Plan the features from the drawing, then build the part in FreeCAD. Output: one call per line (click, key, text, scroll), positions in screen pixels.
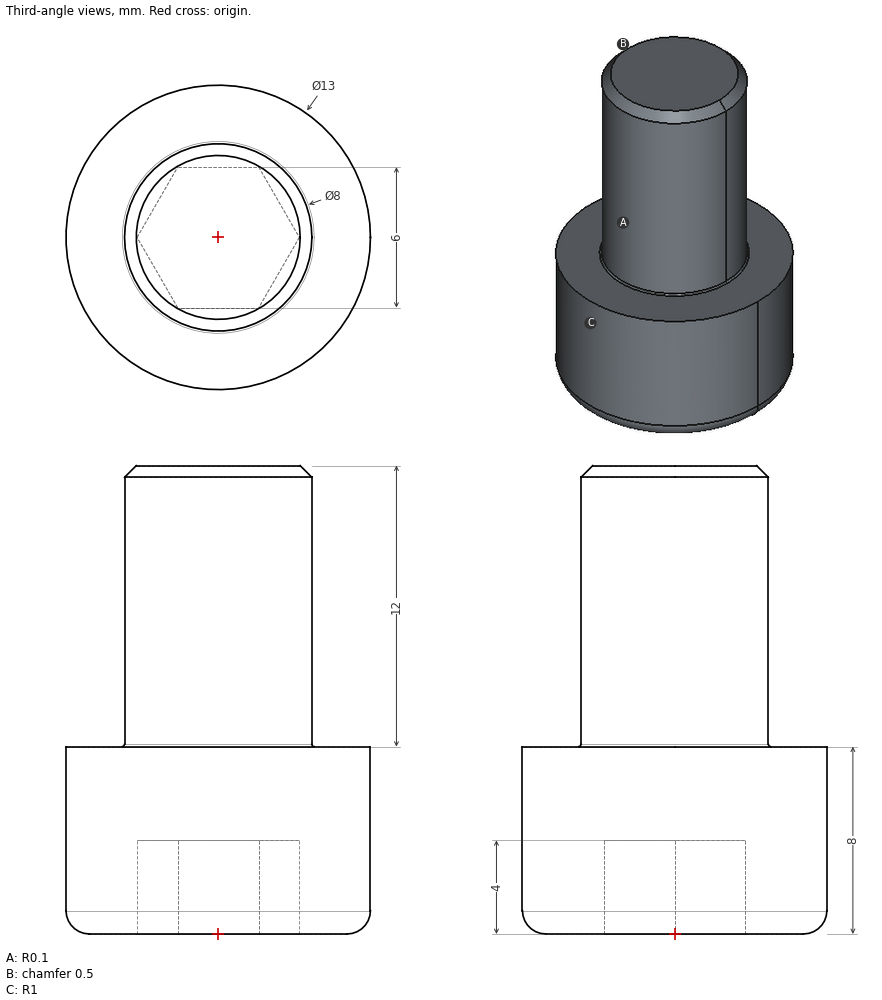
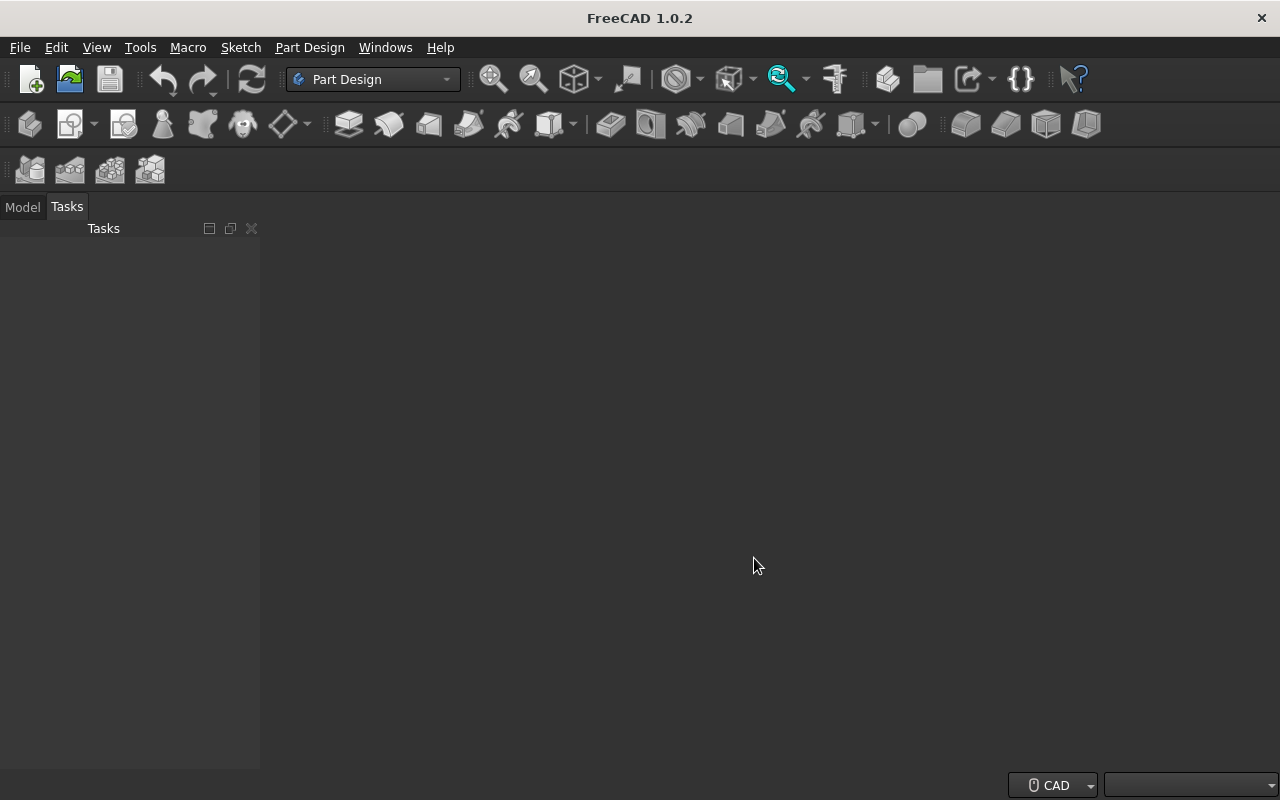
click(30, 80)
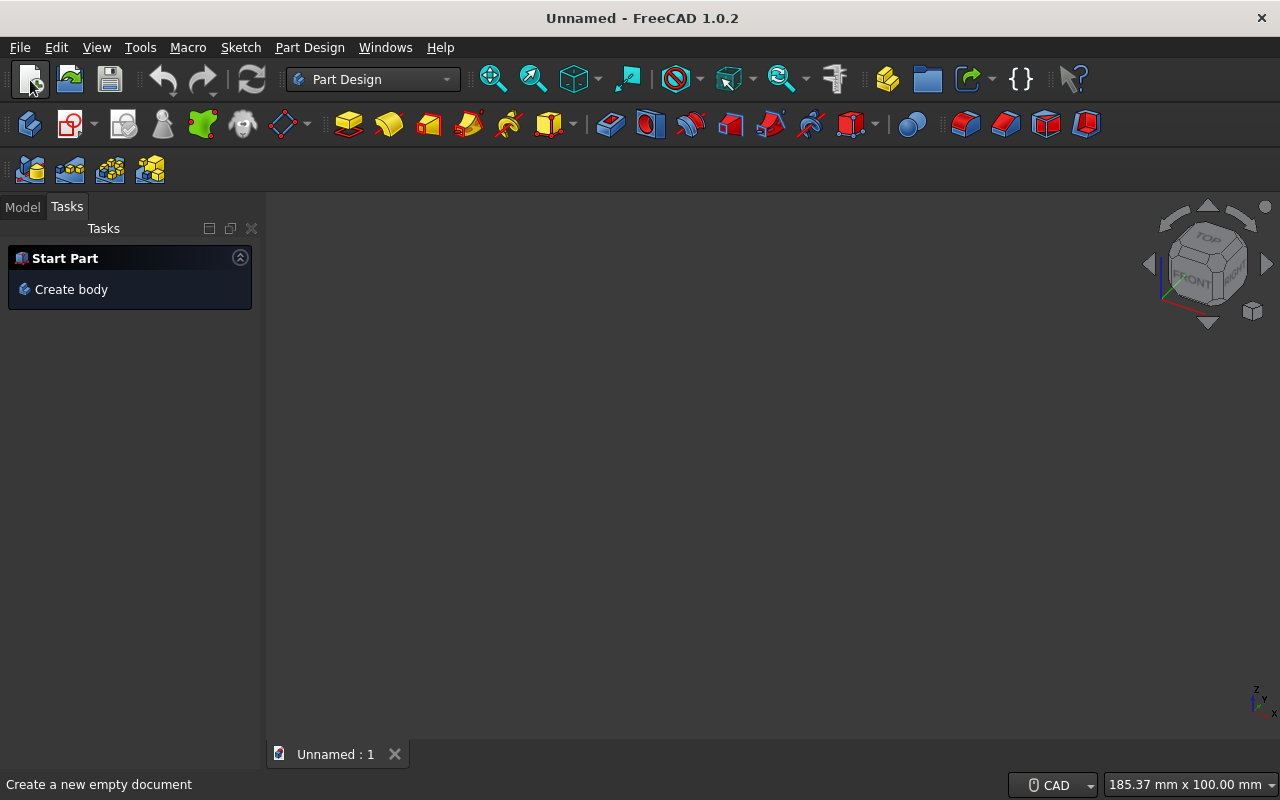
click(70, 124)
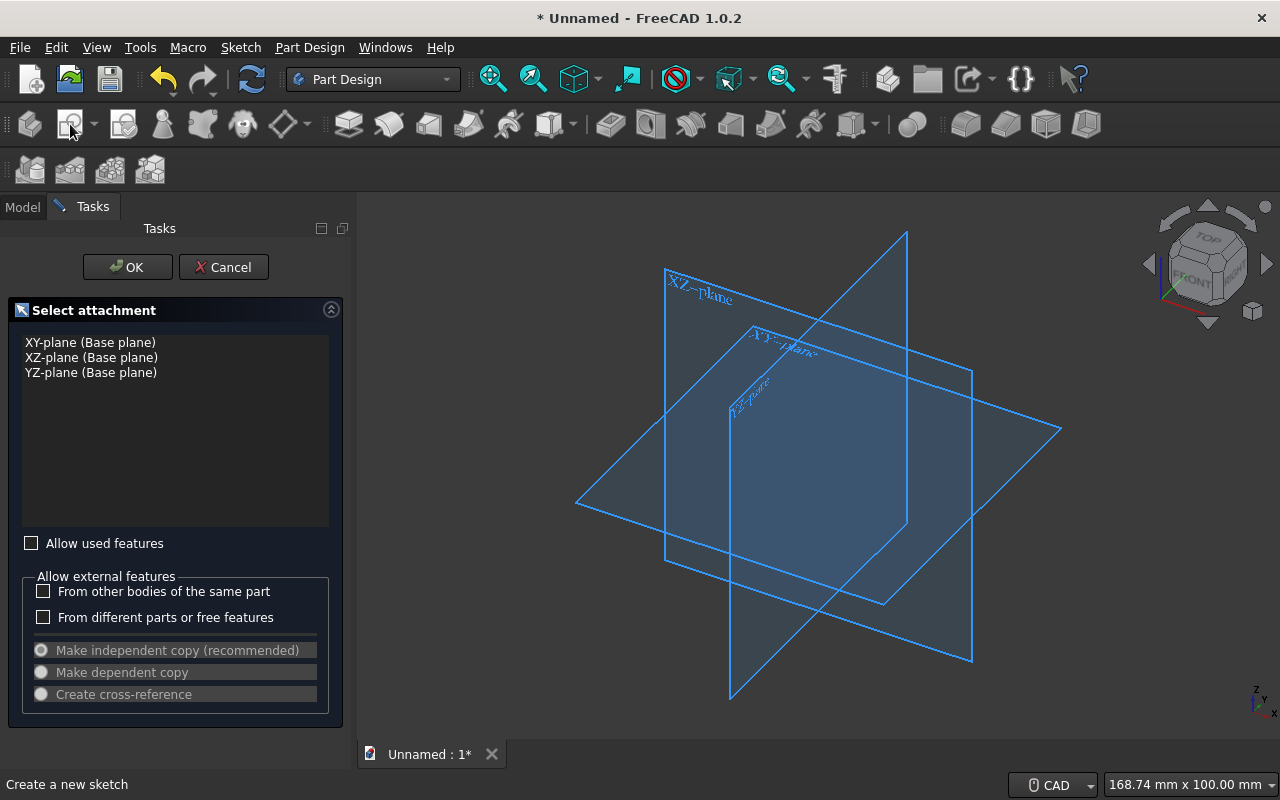
click(82, 342)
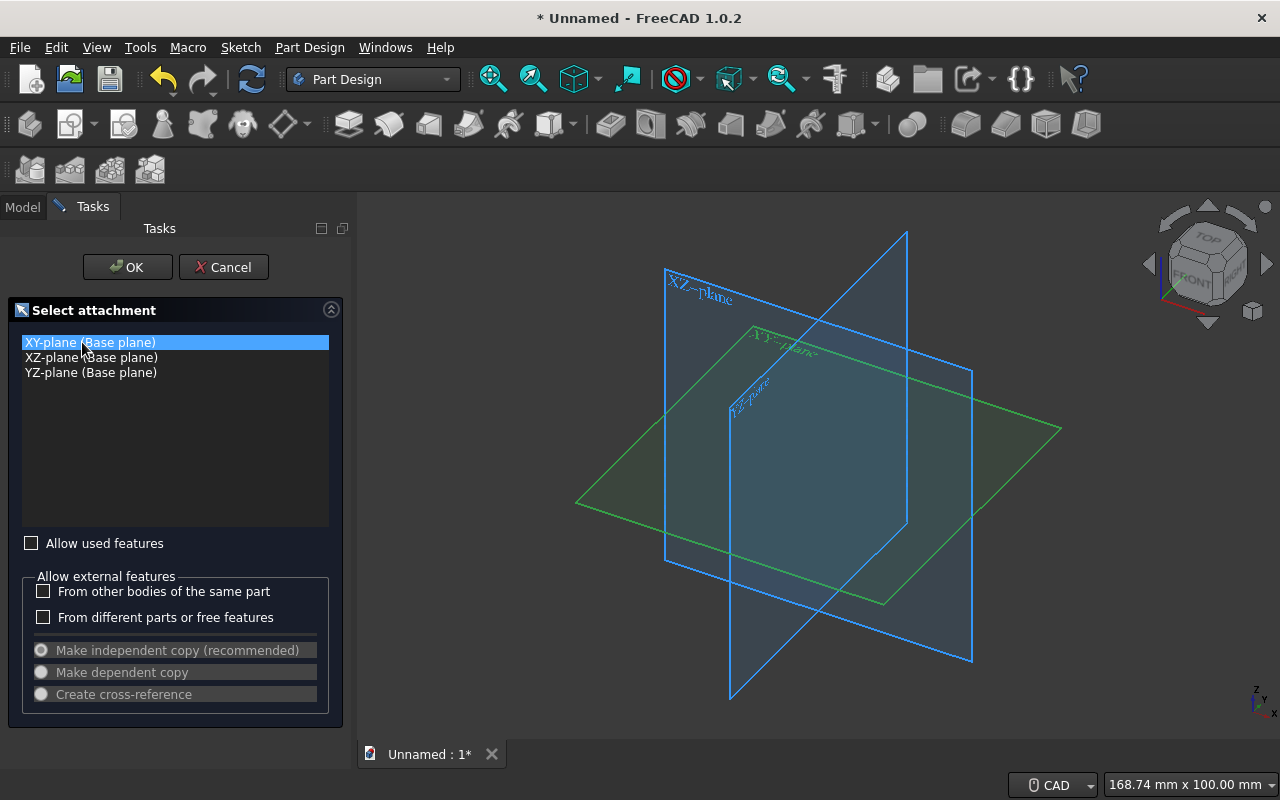
click(128, 267)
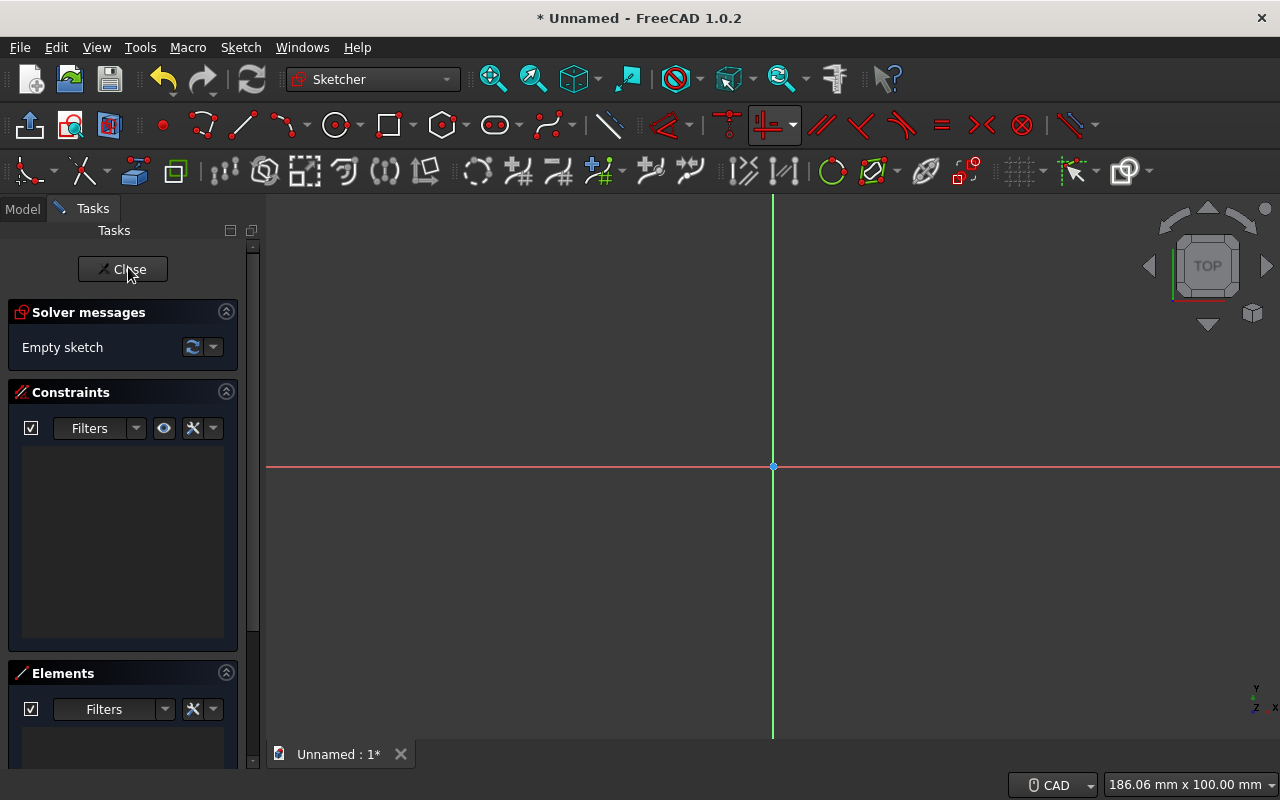
scroll(790, 466, up, 8)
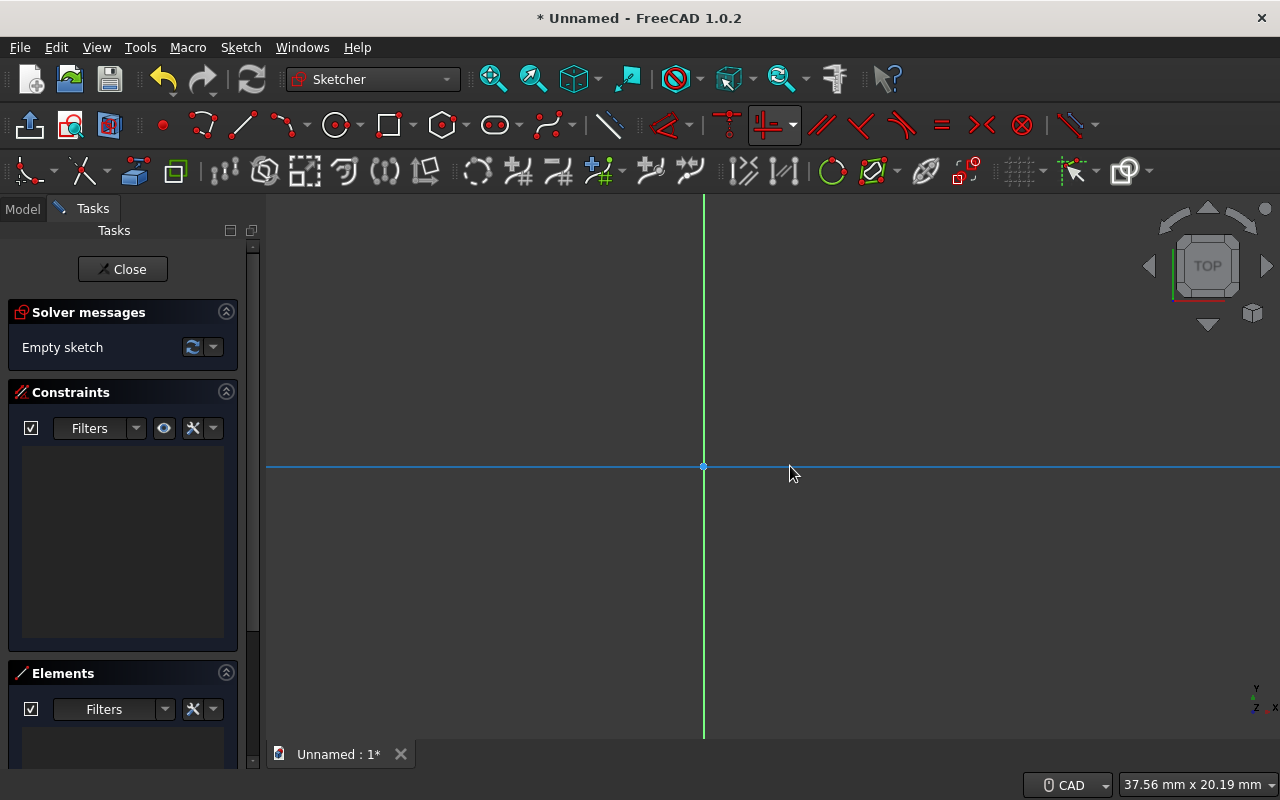
click(336, 126)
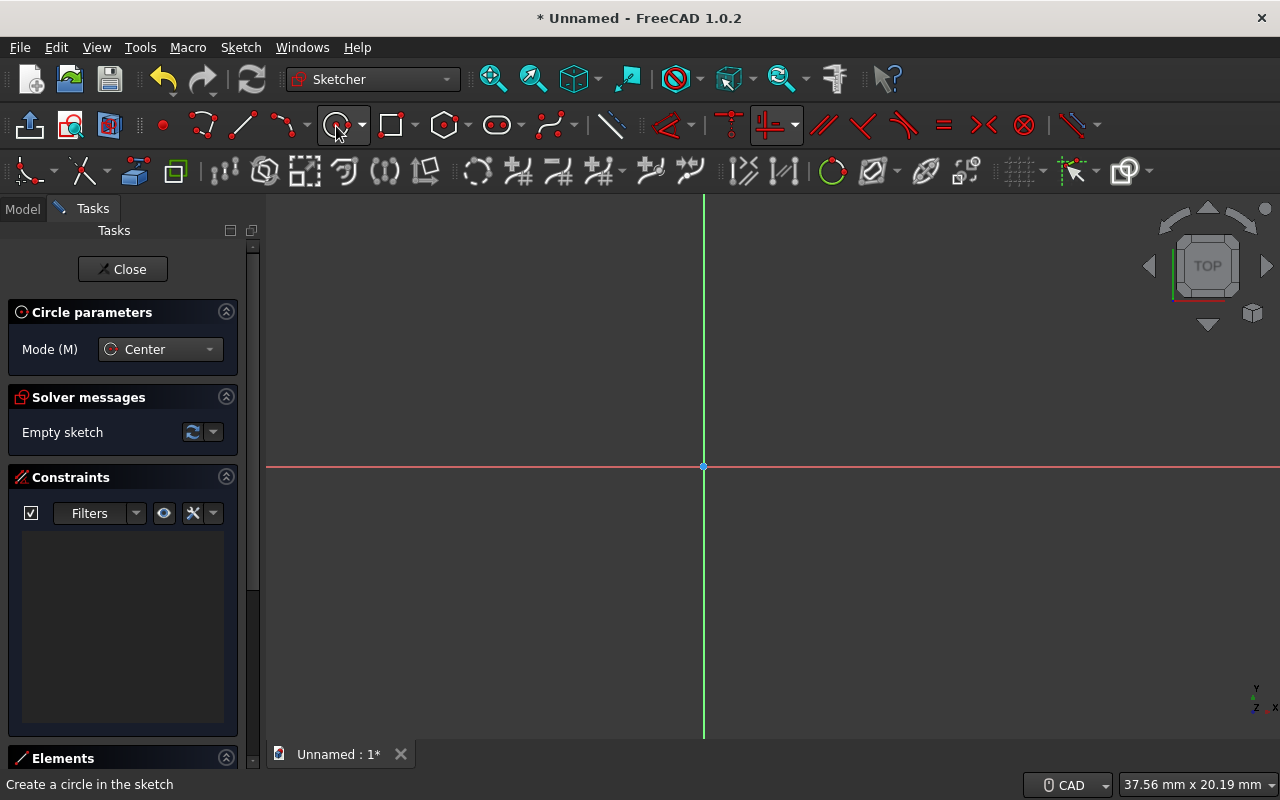
click(704, 466)
click(828, 342)
key(Escape)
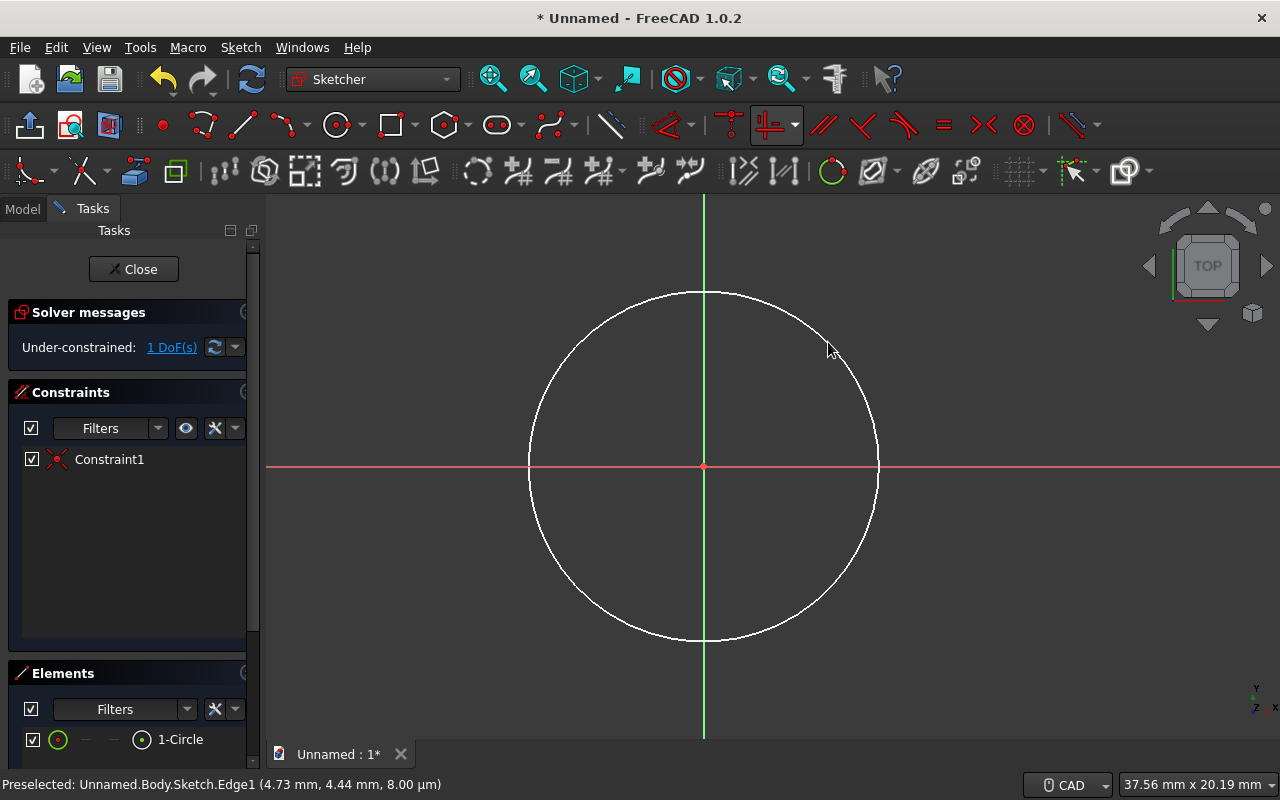
click(827, 342)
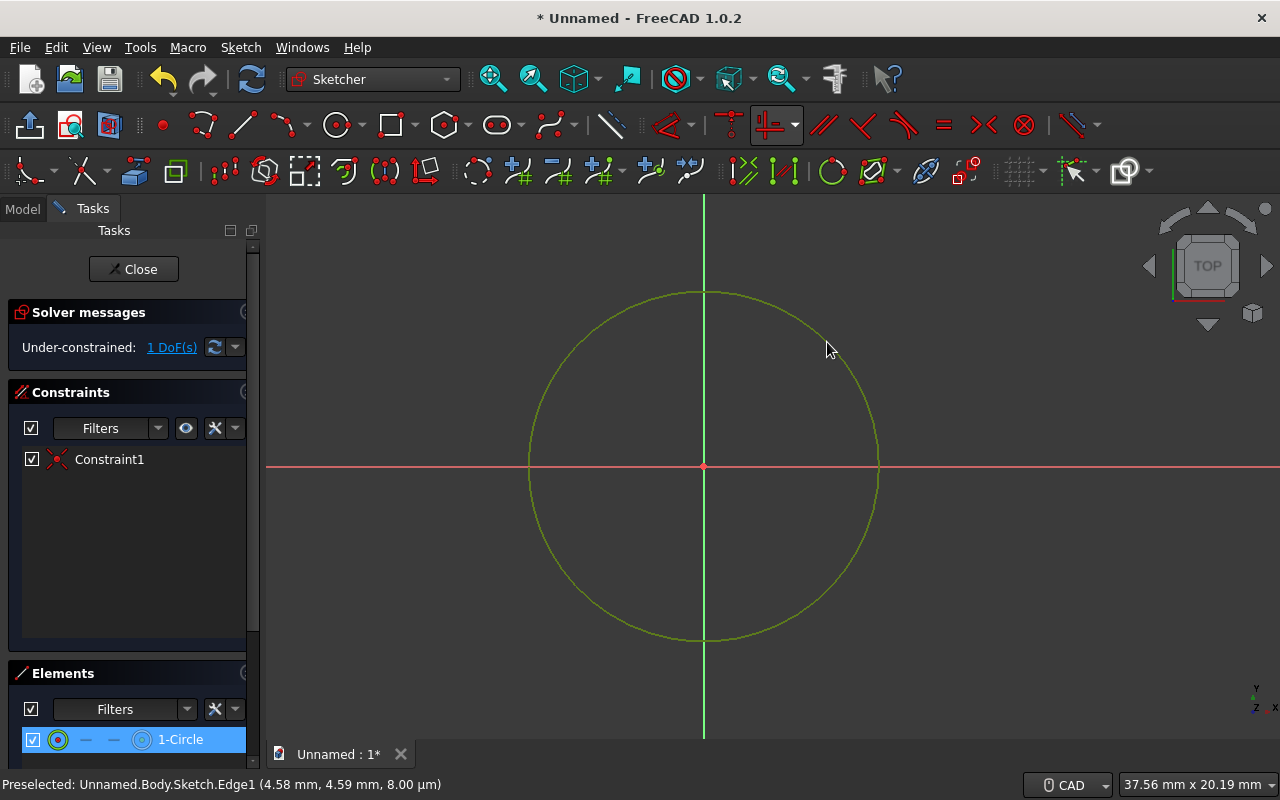
click(694, 126)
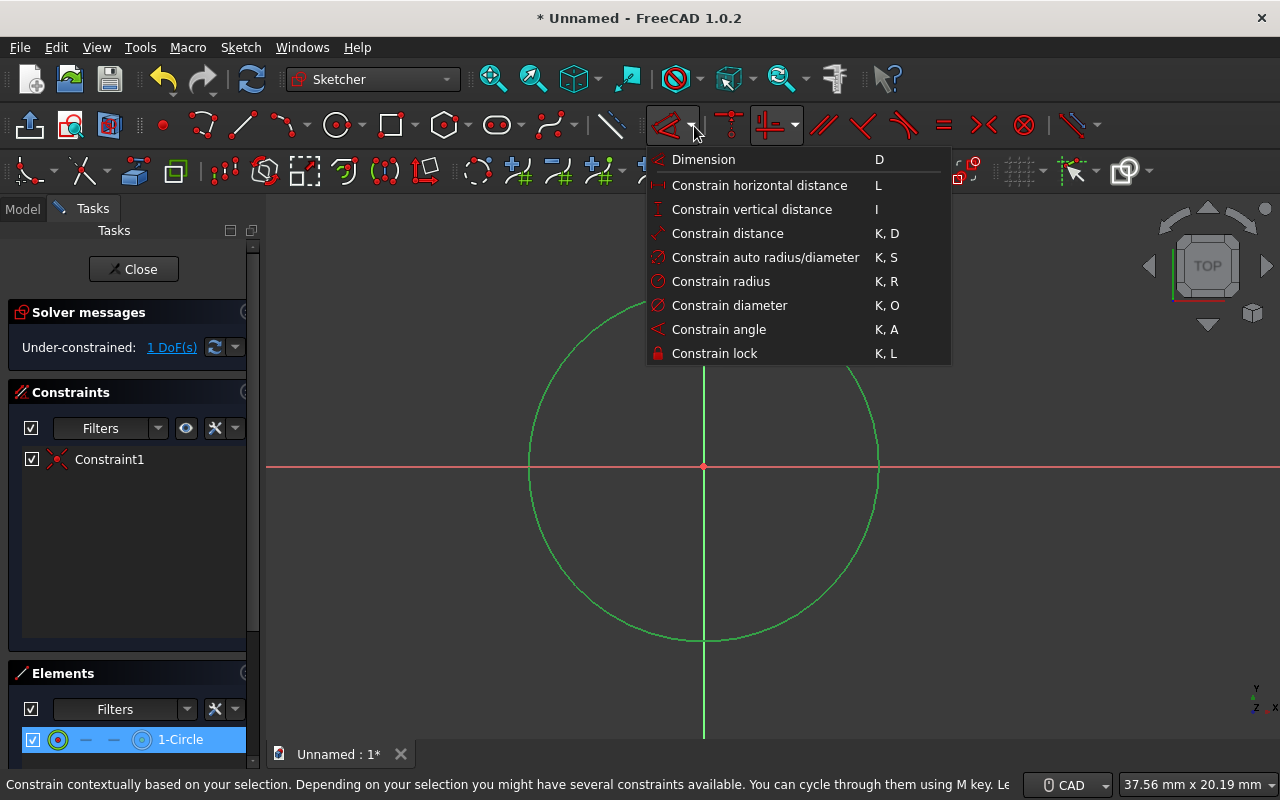
click(799, 305)